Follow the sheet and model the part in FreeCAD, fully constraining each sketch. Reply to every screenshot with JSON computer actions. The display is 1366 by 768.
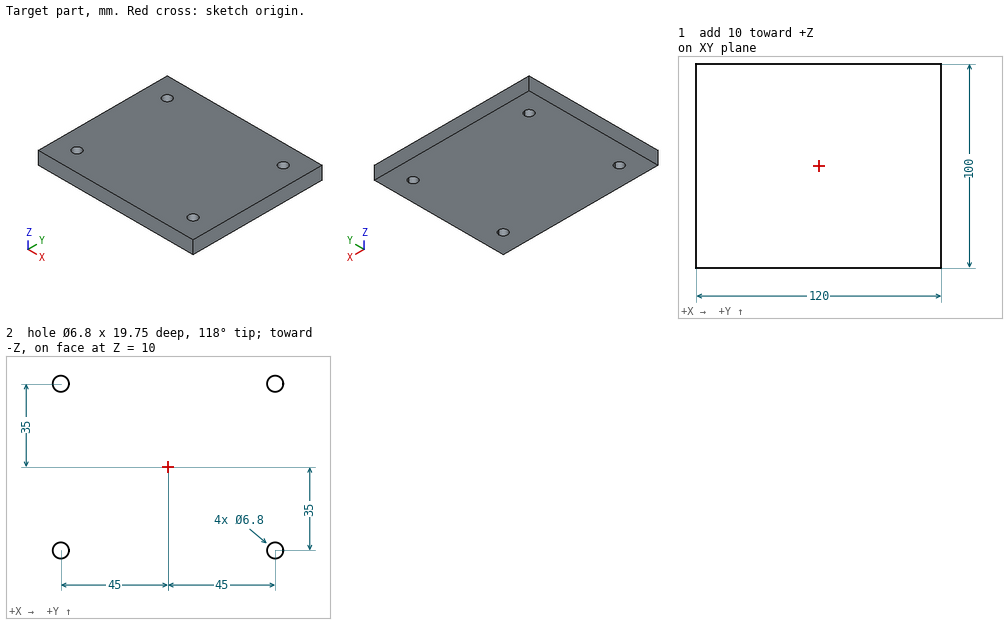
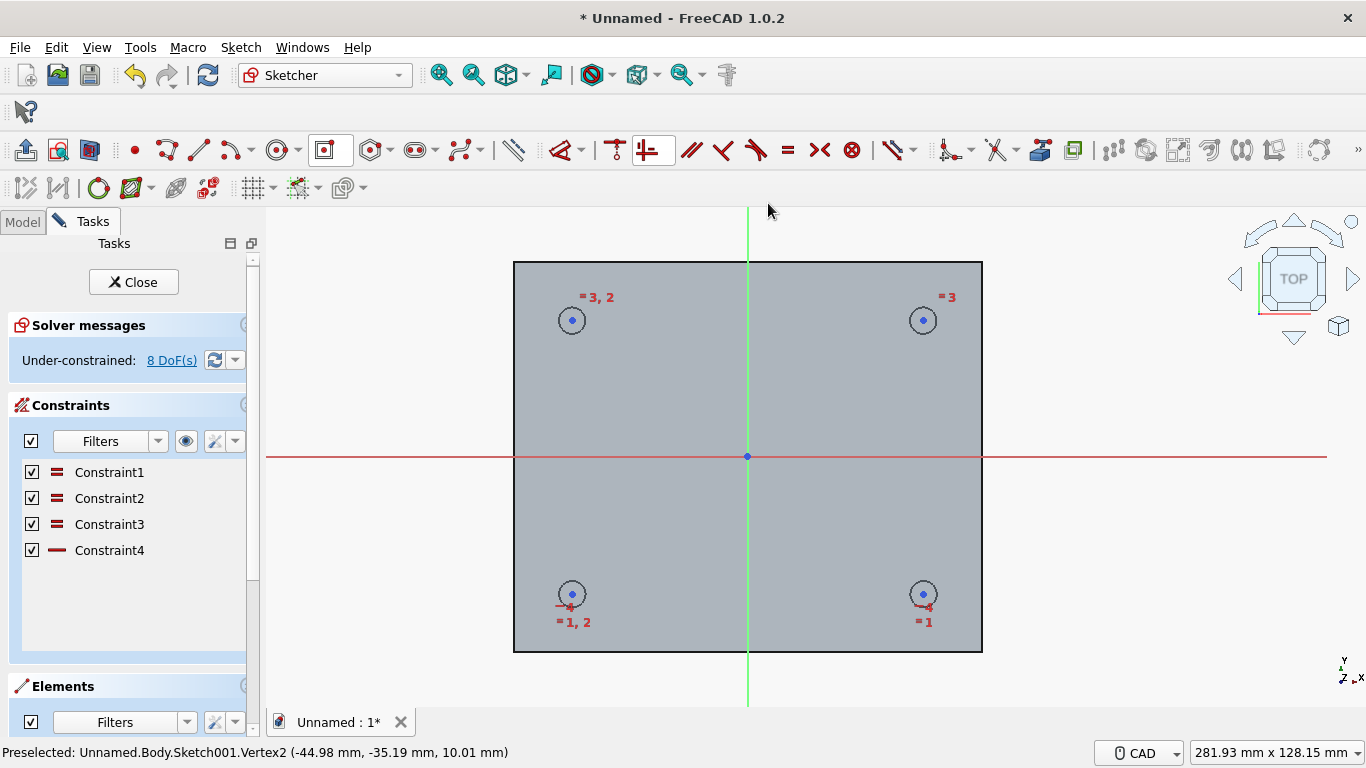
{"action": "left_click", "coordinate": [572, 594]}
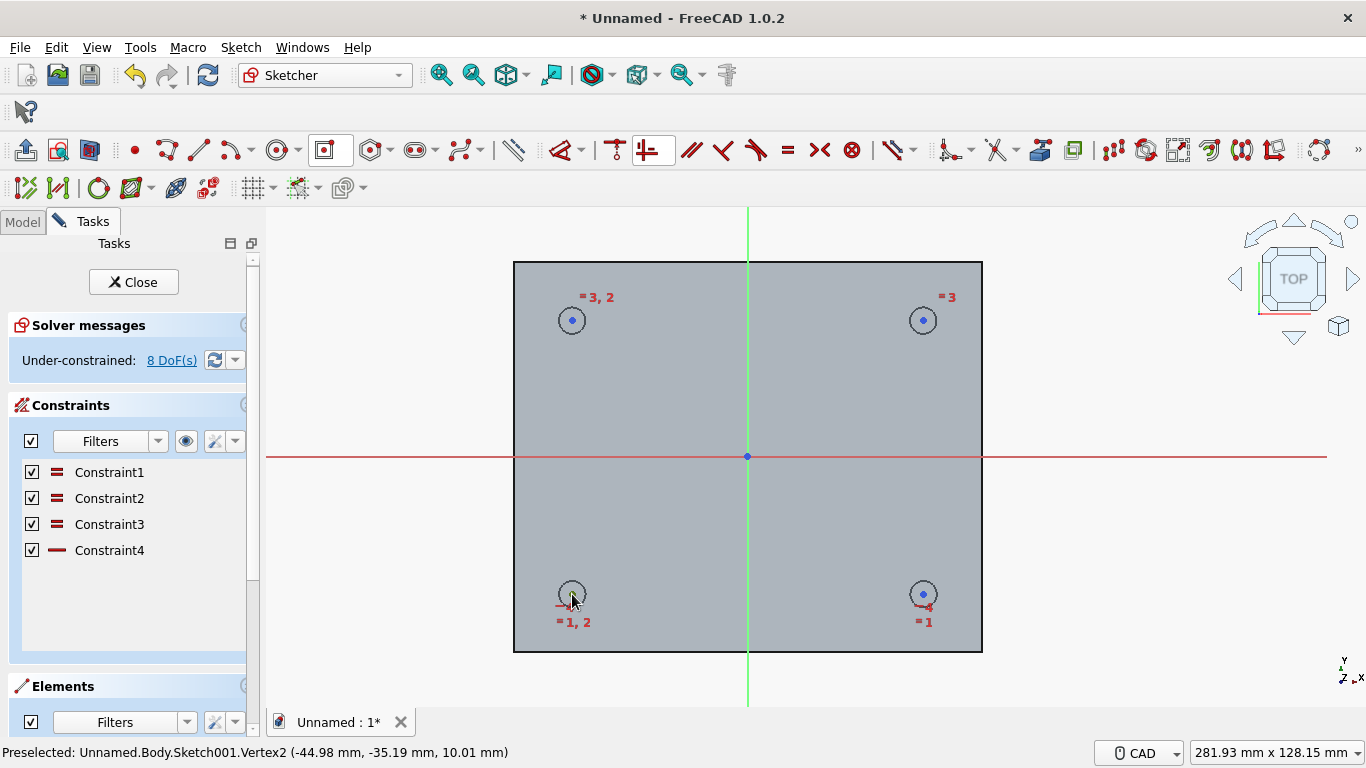
{"action": "left_click", "coordinate": [572, 321]}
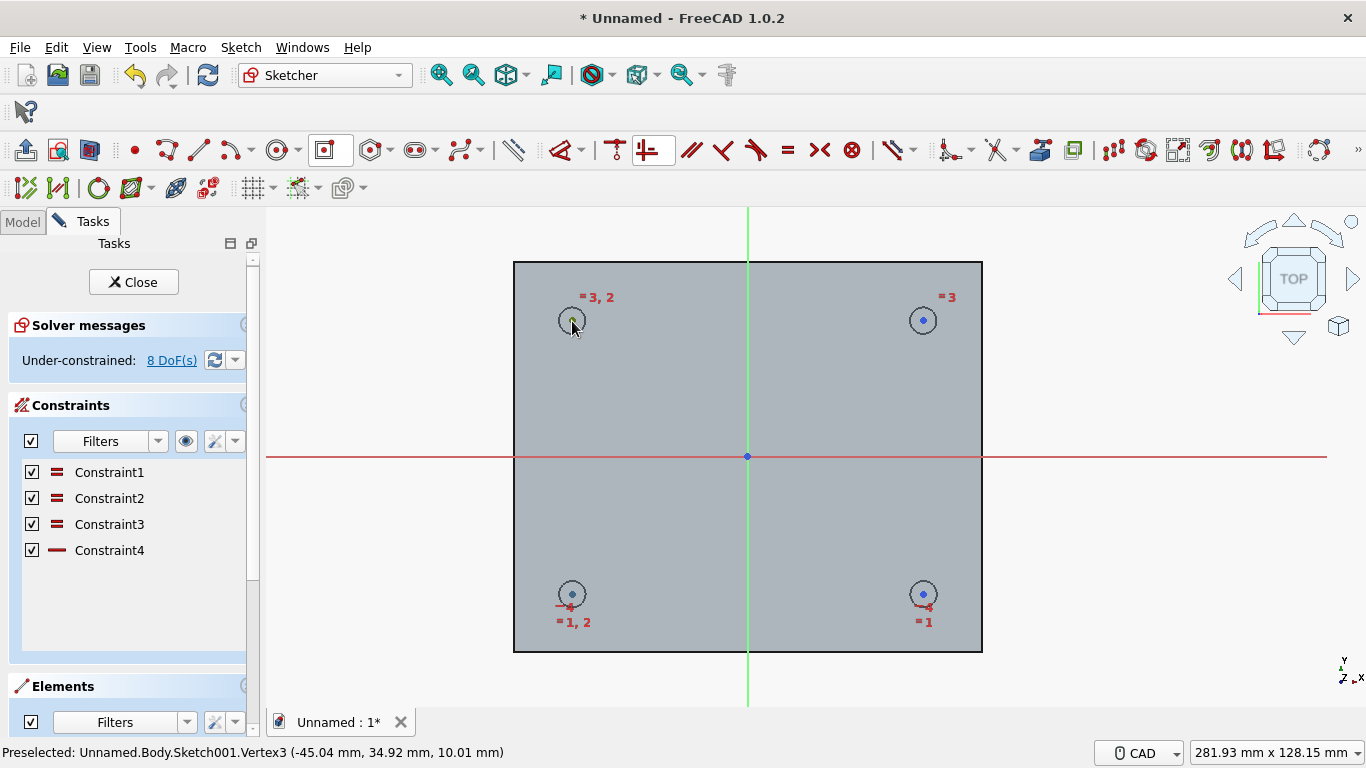
{"action": "left_click", "coordinate": [670, 150]}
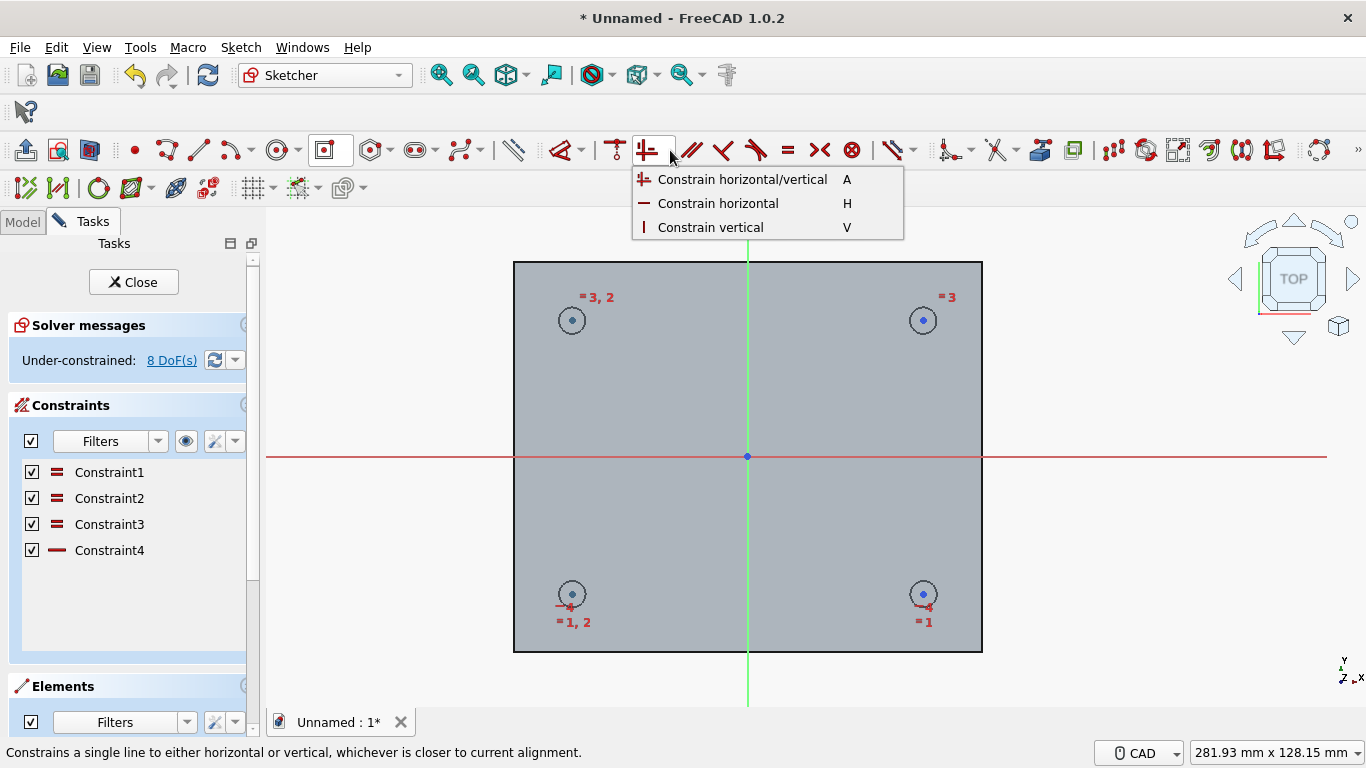
{"action": "left_click", "coordinate": [768, 227]}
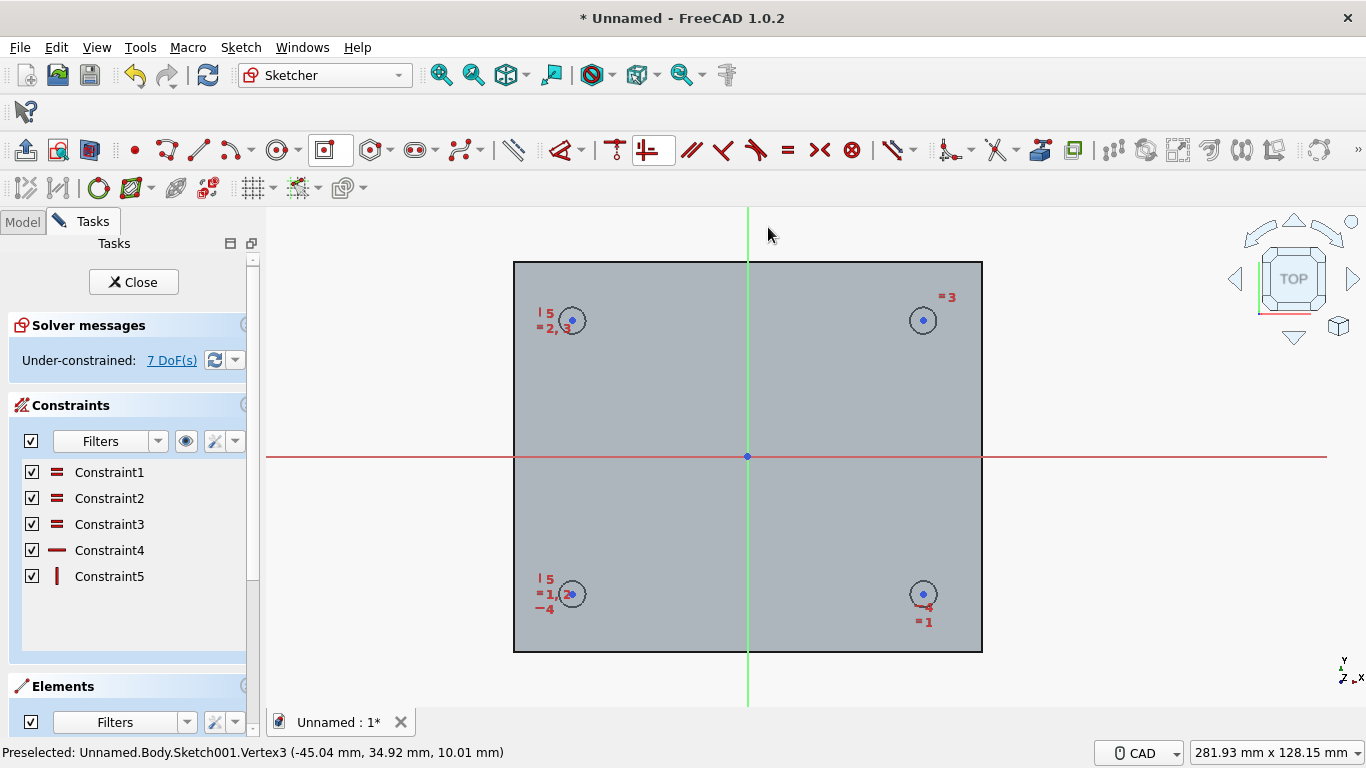
{"action": "left_click", "coordinate": [924, 594]}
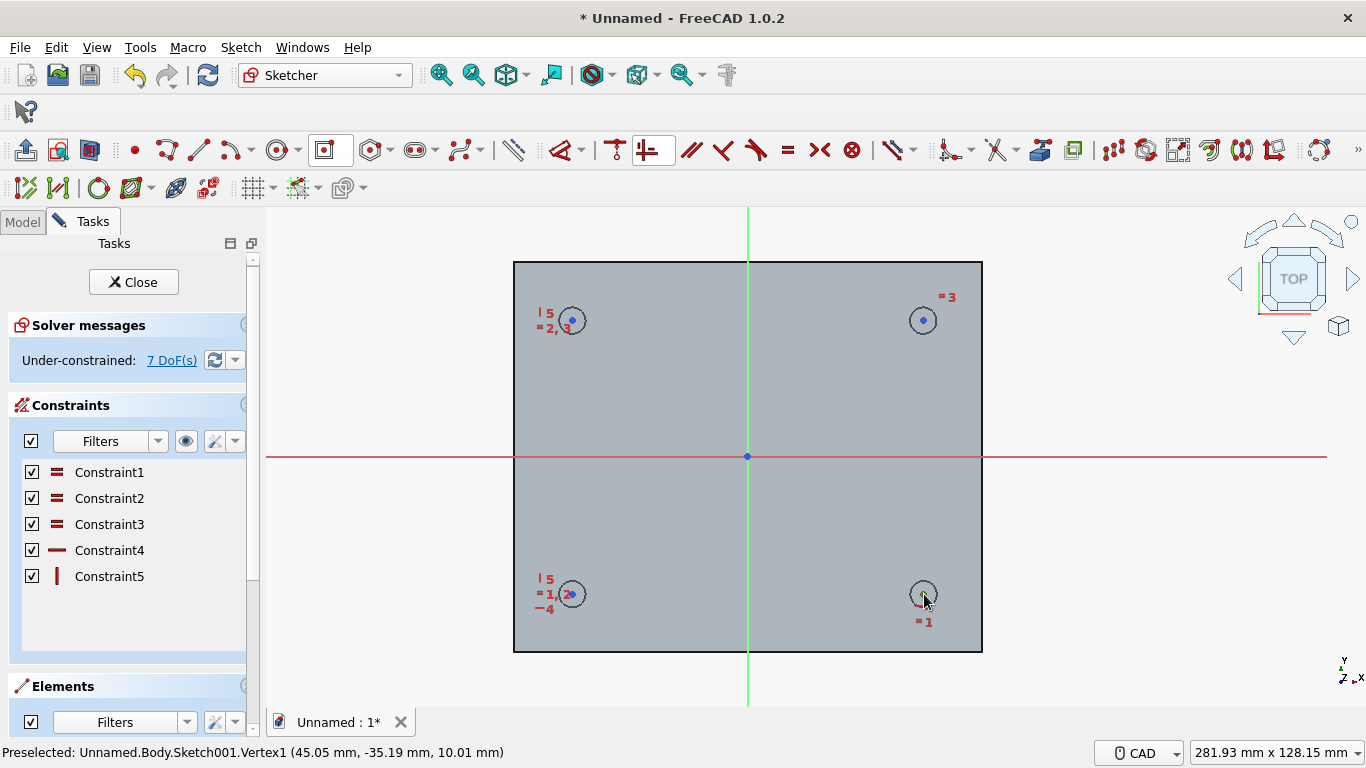
{"action": "left_click", "coordinate": [923, 321]}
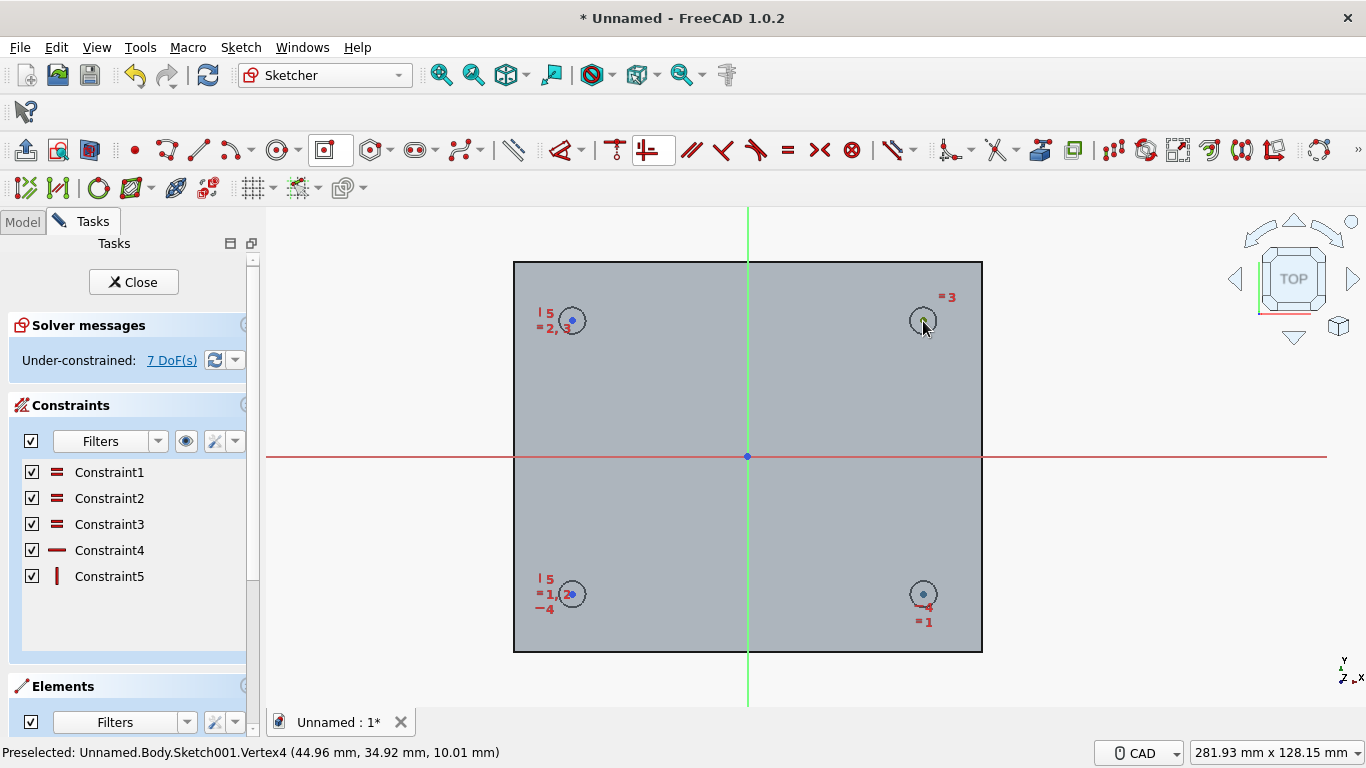
{"action": "key", "text": "v"}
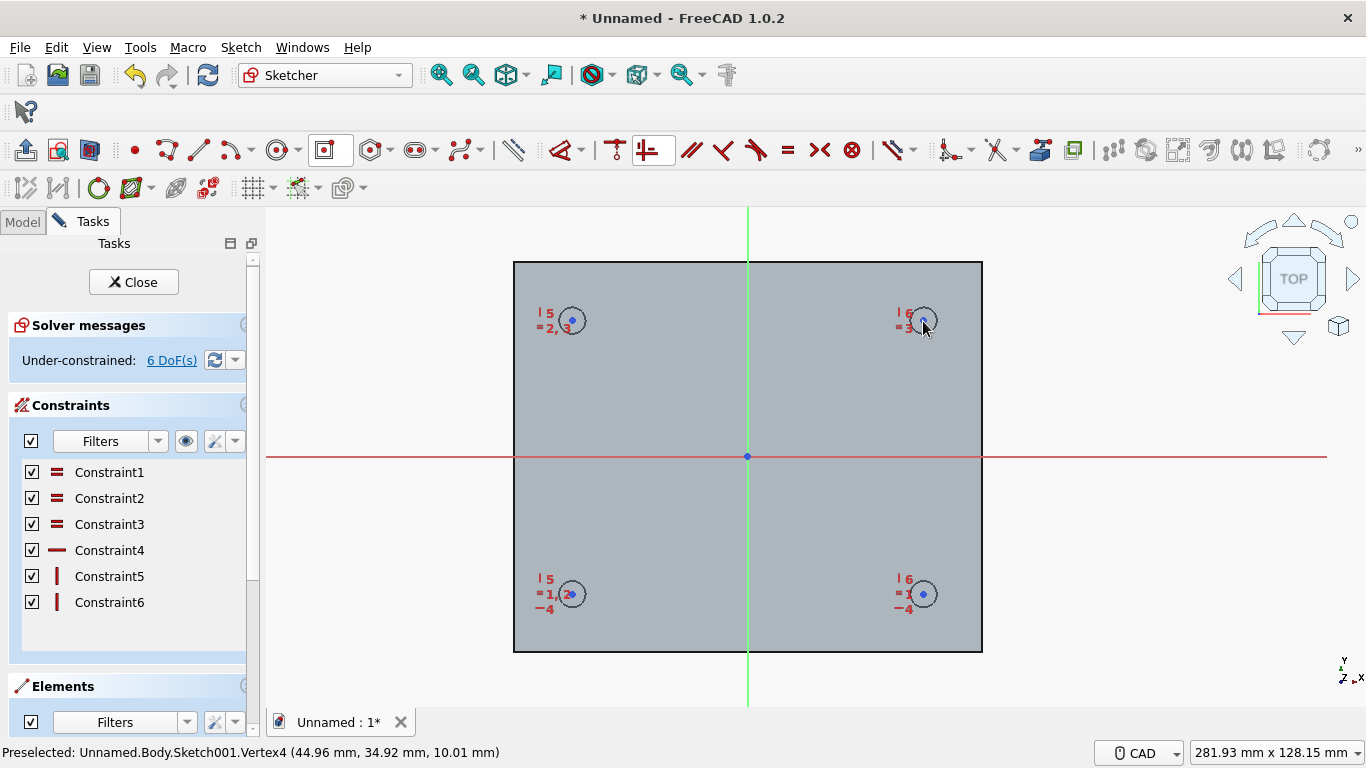
{"action": "left_click", "coordinate": [572, 321]}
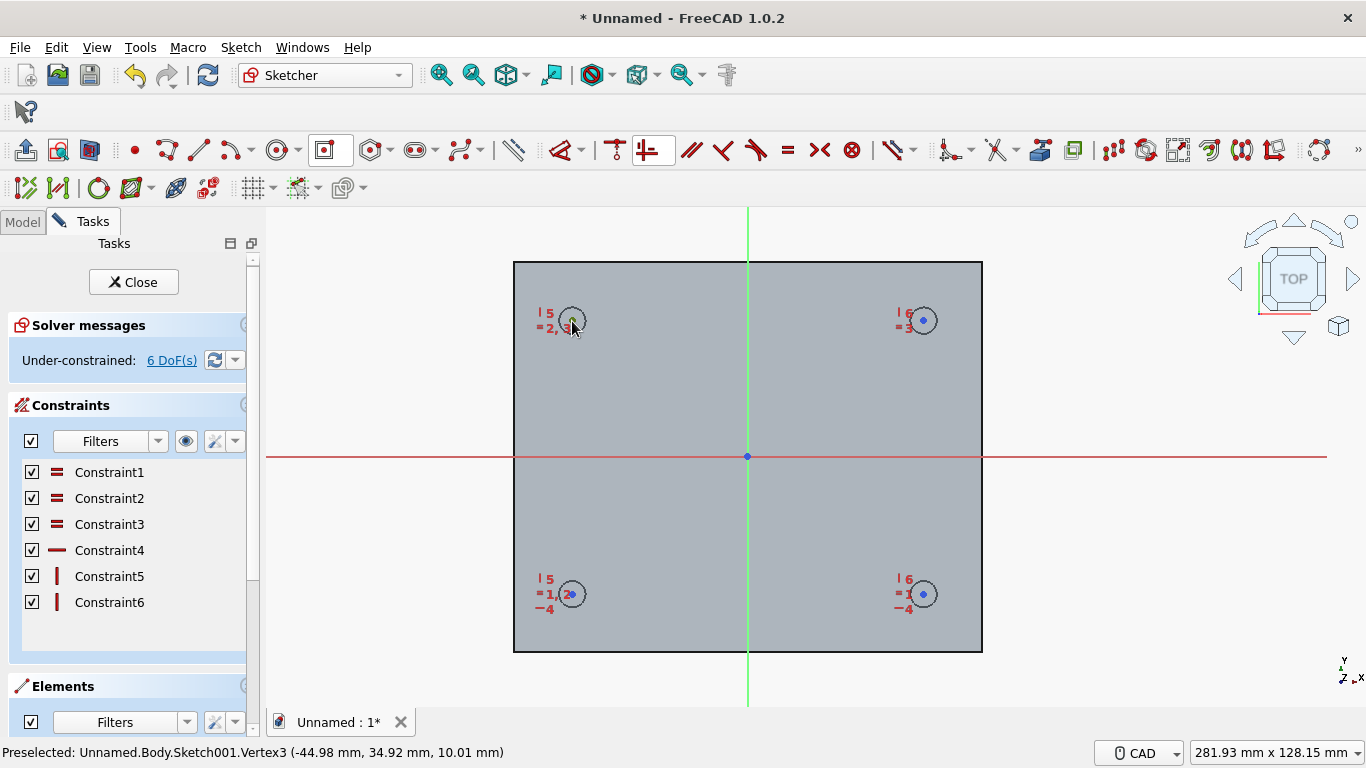
{"action": "left_click", "coordinate": [924, 321]}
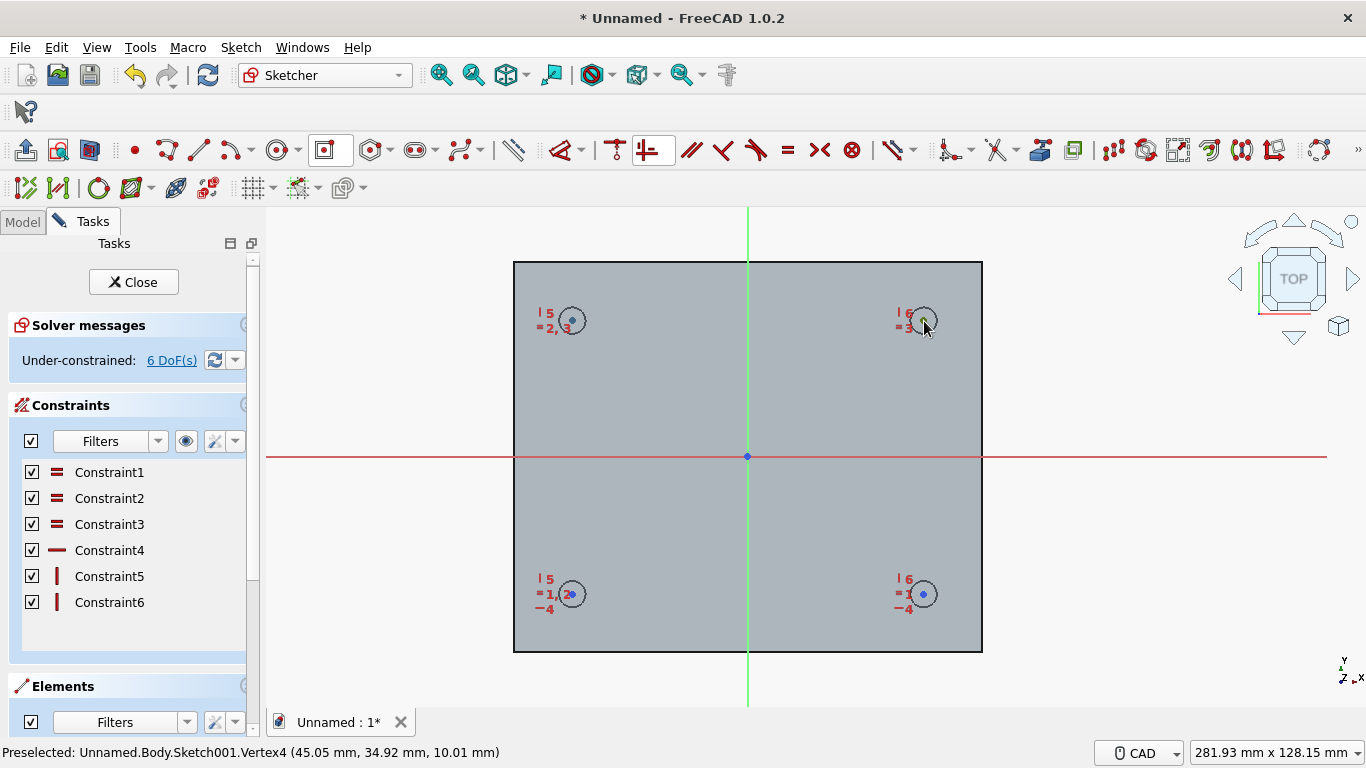
{"action": "key", "text": "h"}